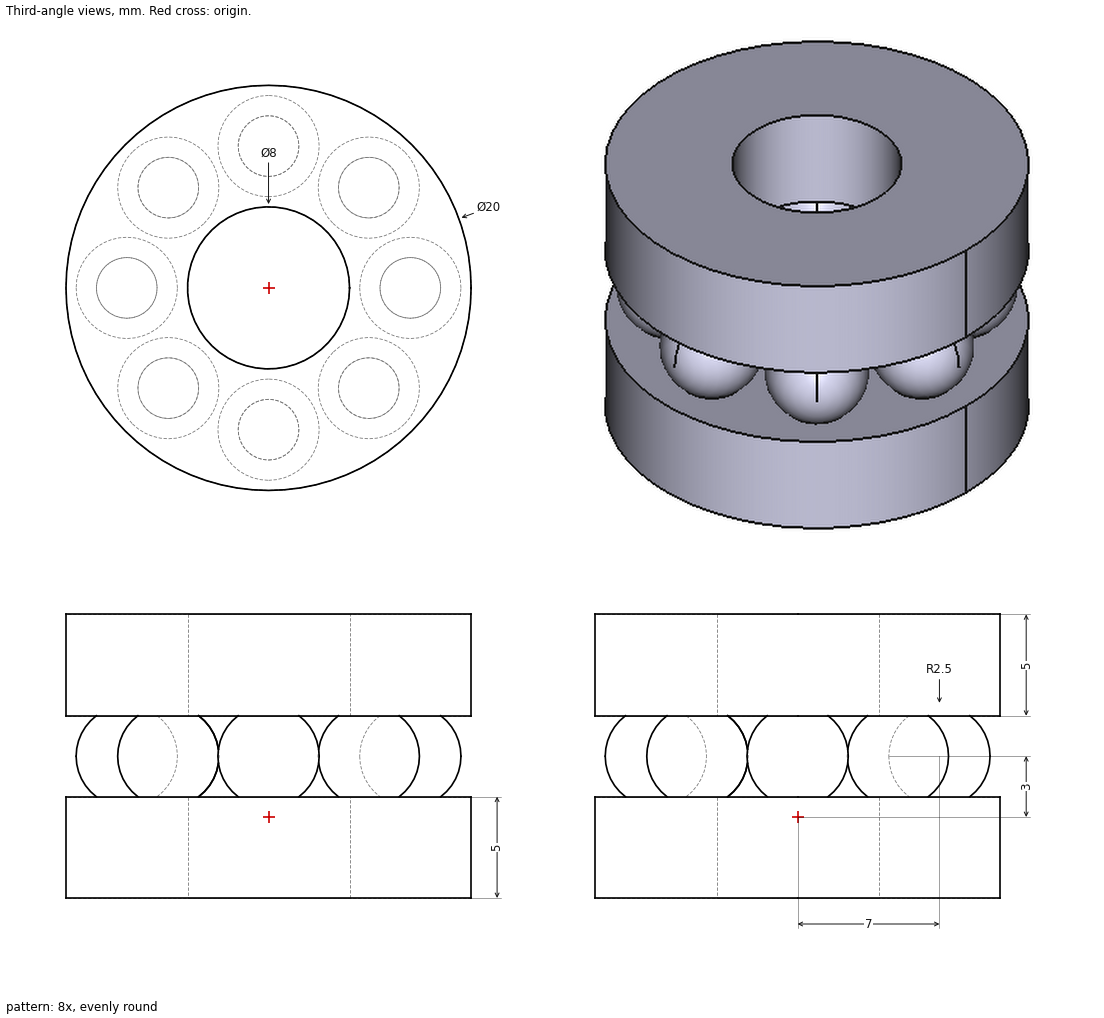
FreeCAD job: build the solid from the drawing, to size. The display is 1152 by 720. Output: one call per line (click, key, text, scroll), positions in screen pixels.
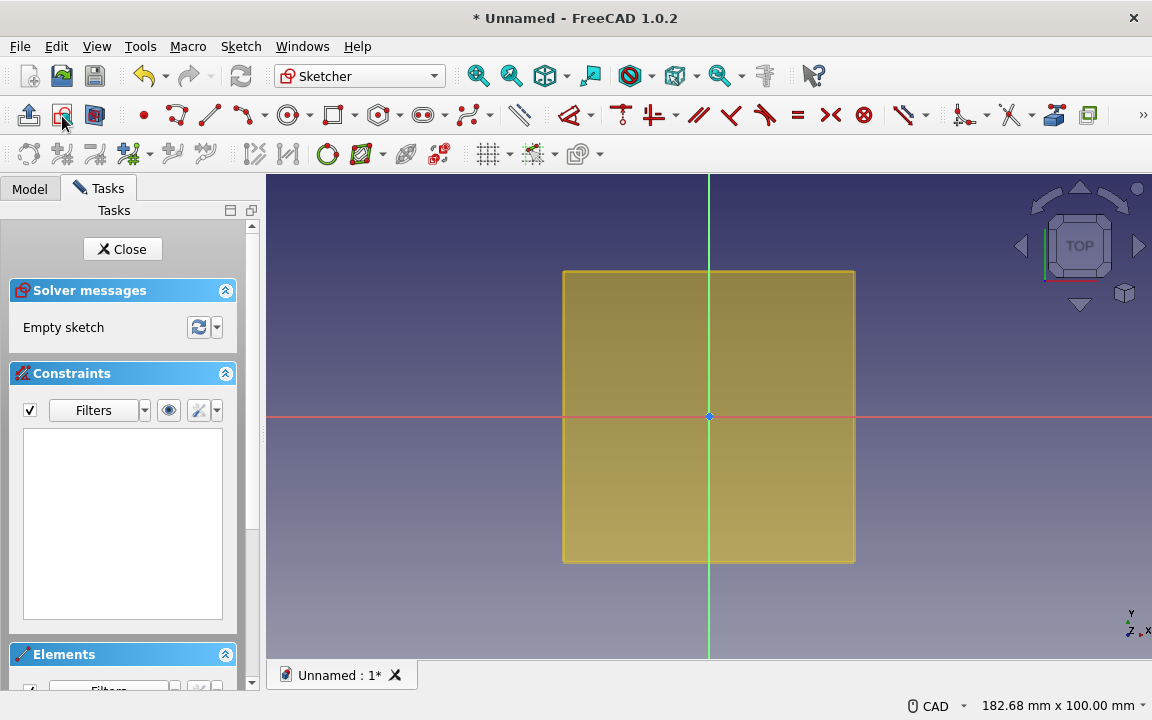
scroll(739, 416, up, 6)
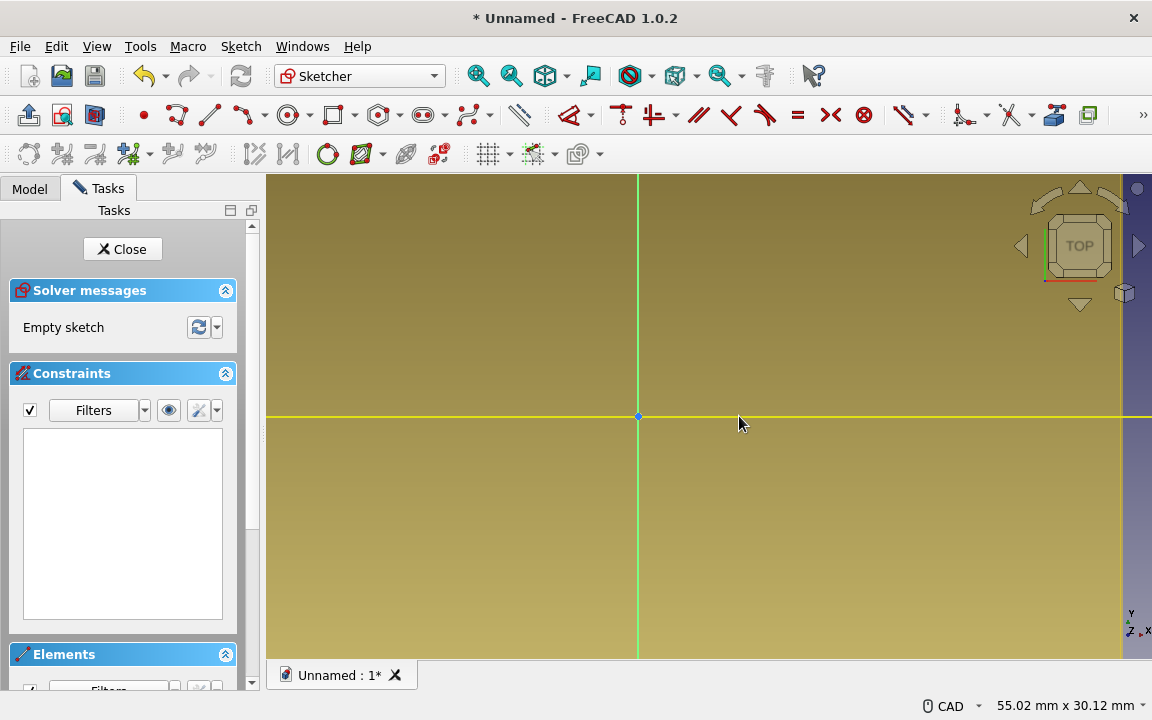
click(288, 116)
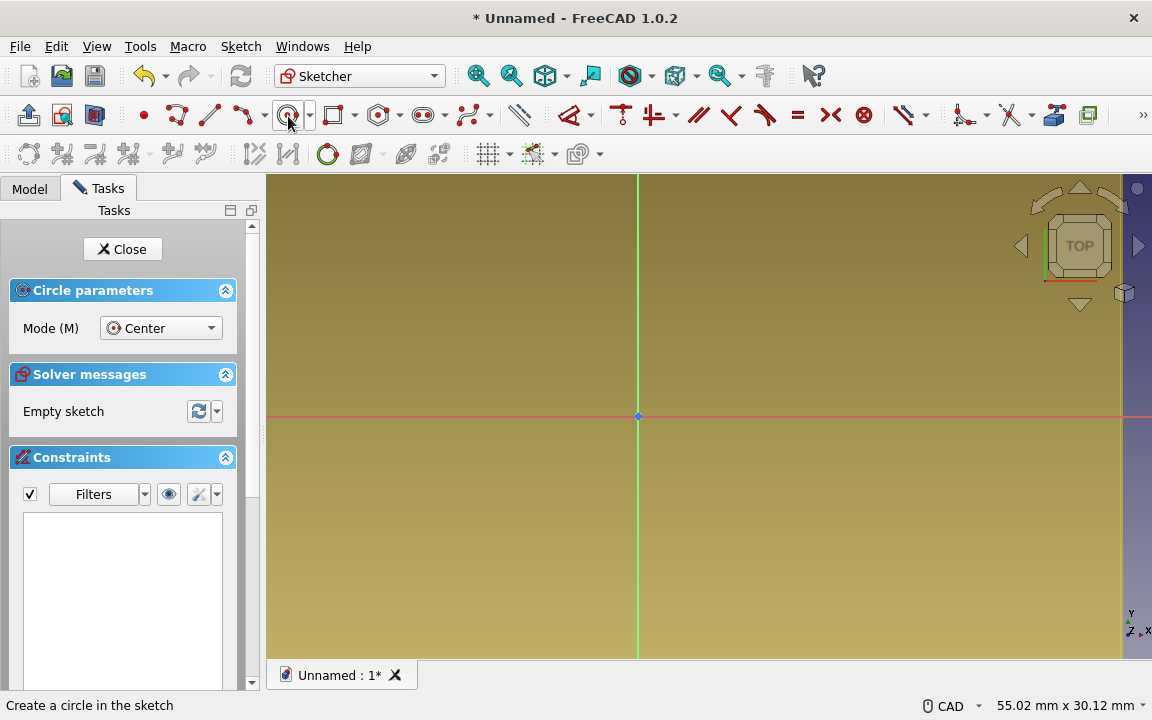
click(638, 416)
click(752, 303)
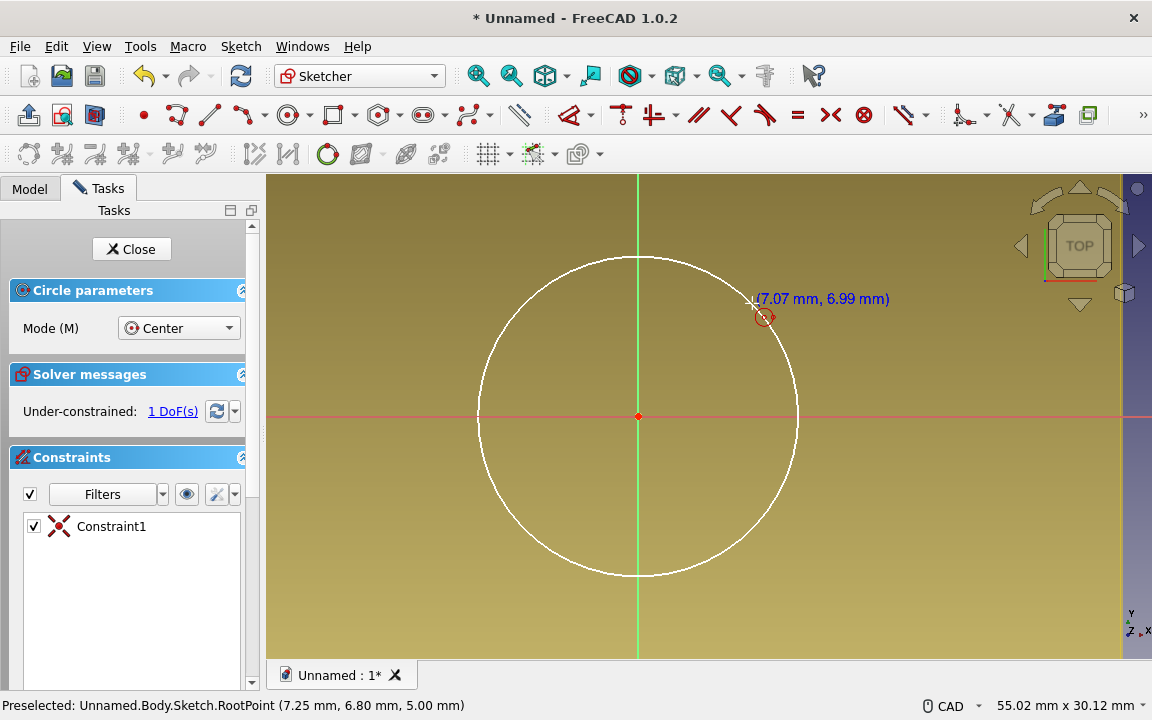
click(638, 416)
click(684, 371)
key(Escape)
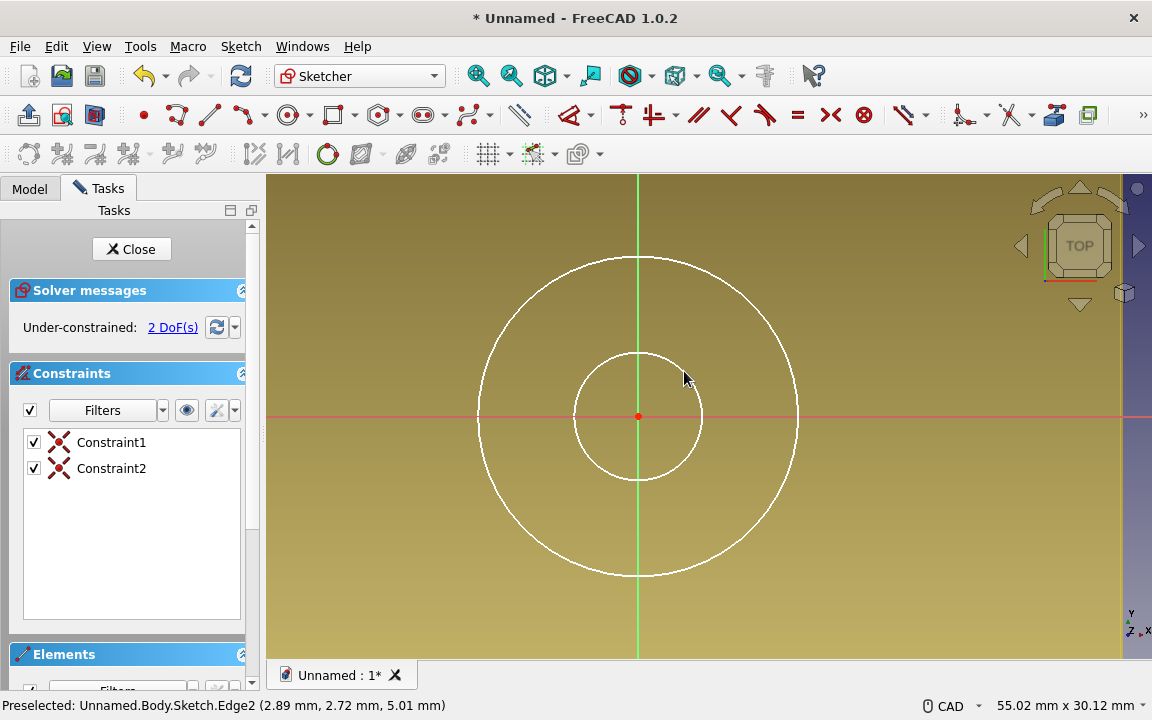
click(568, 116)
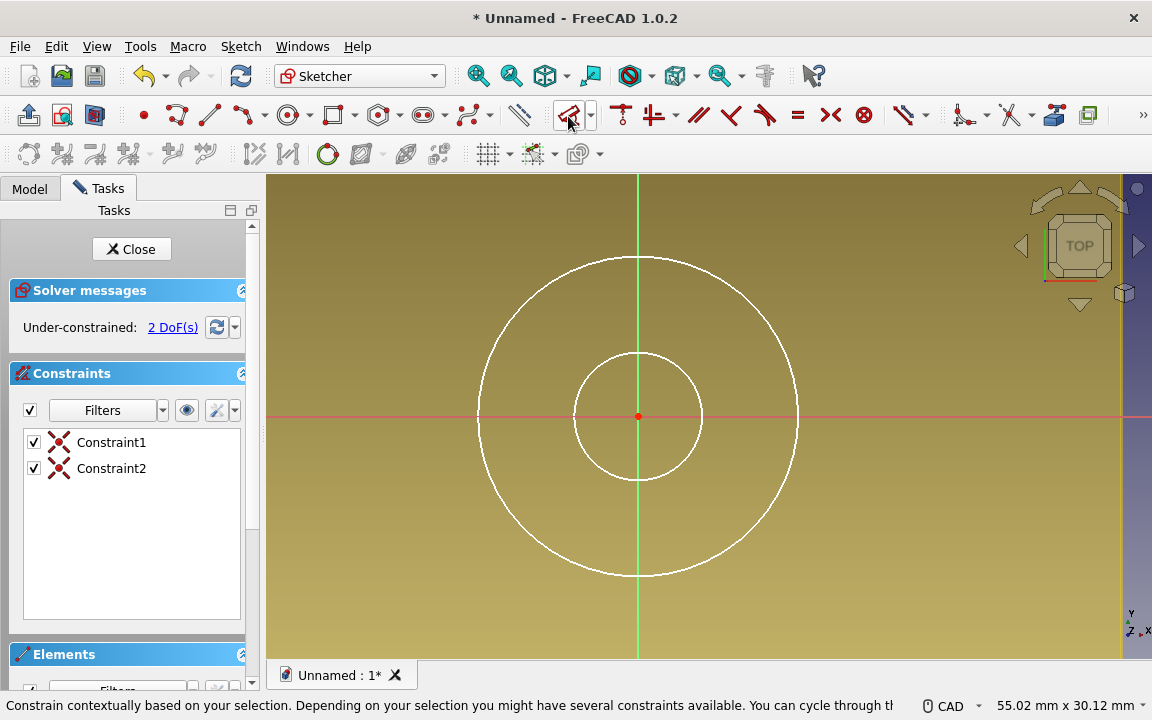
click(751, 303)
click(774, 280)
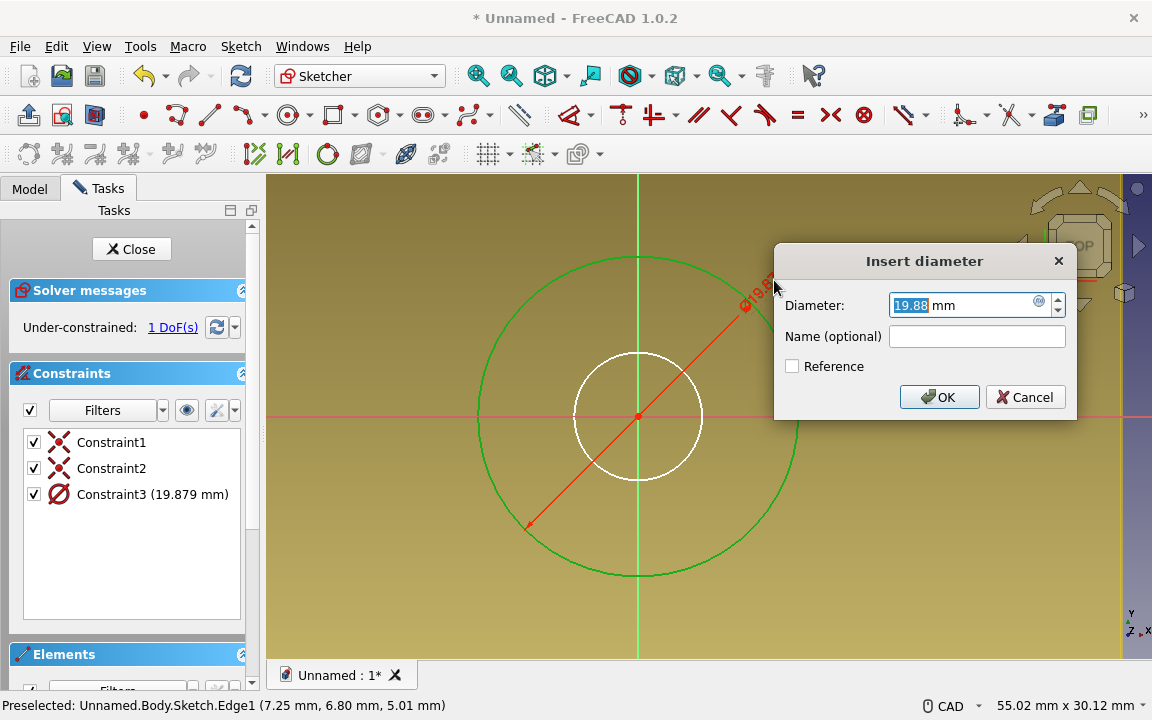
text(20)
key(Return)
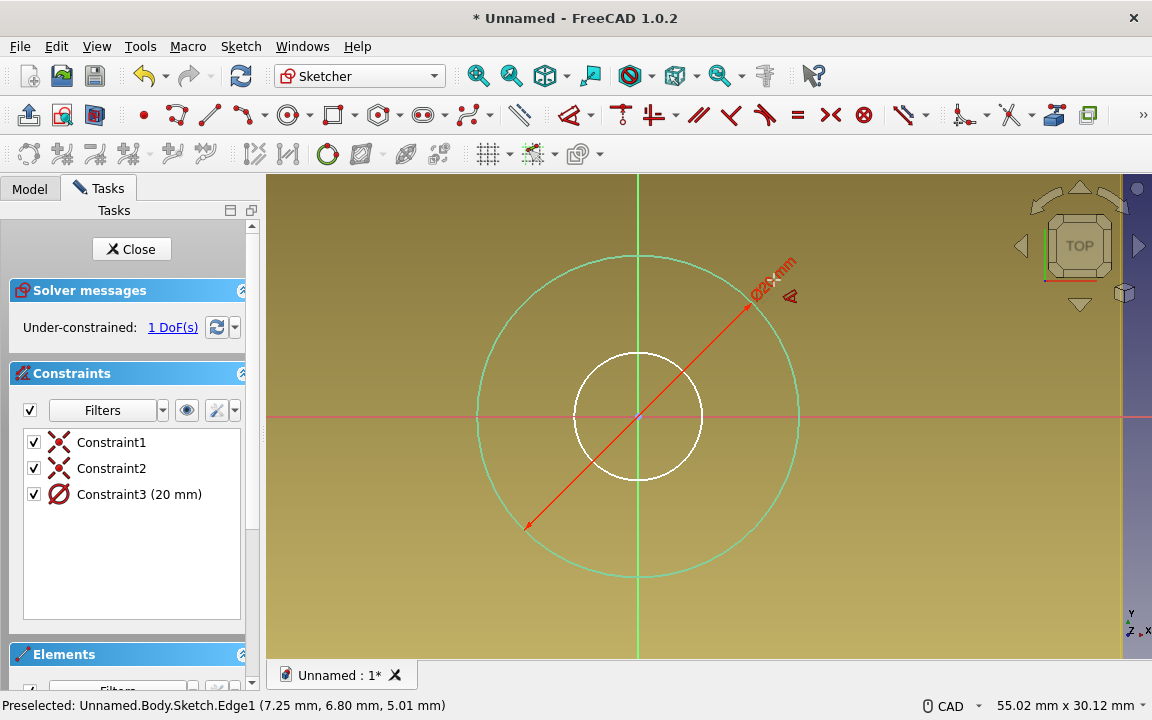
click(683, 371)
click(705, 348)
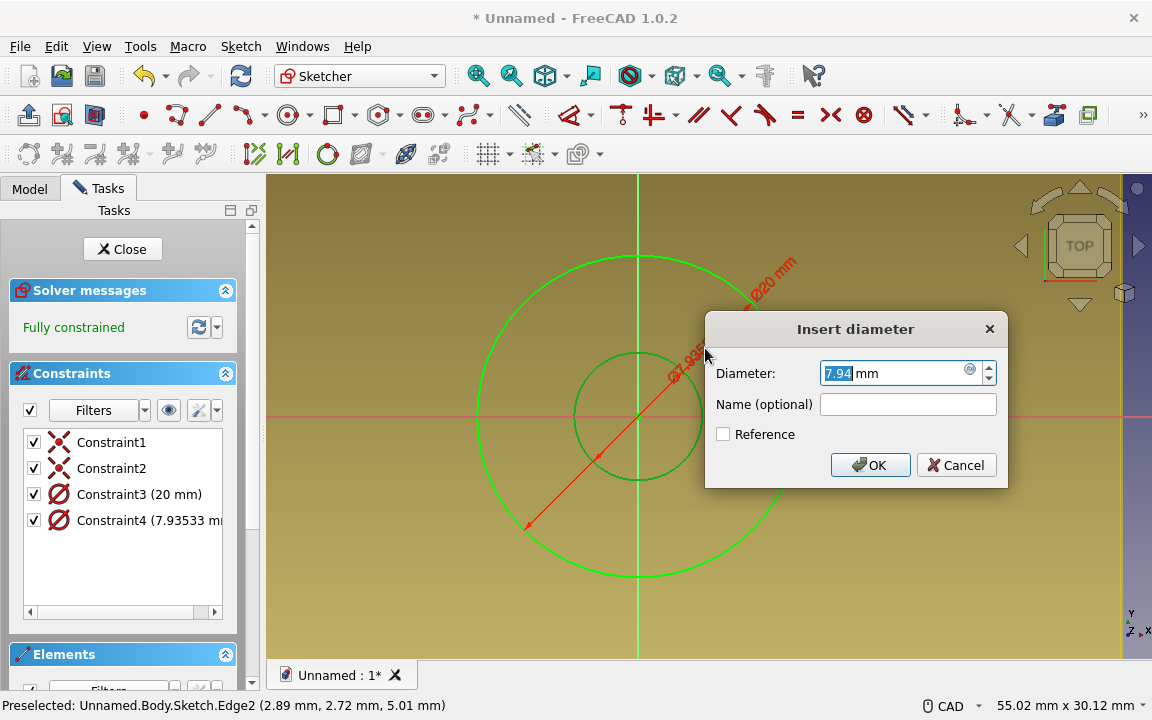
text(8)
key(Return)
key(Escape)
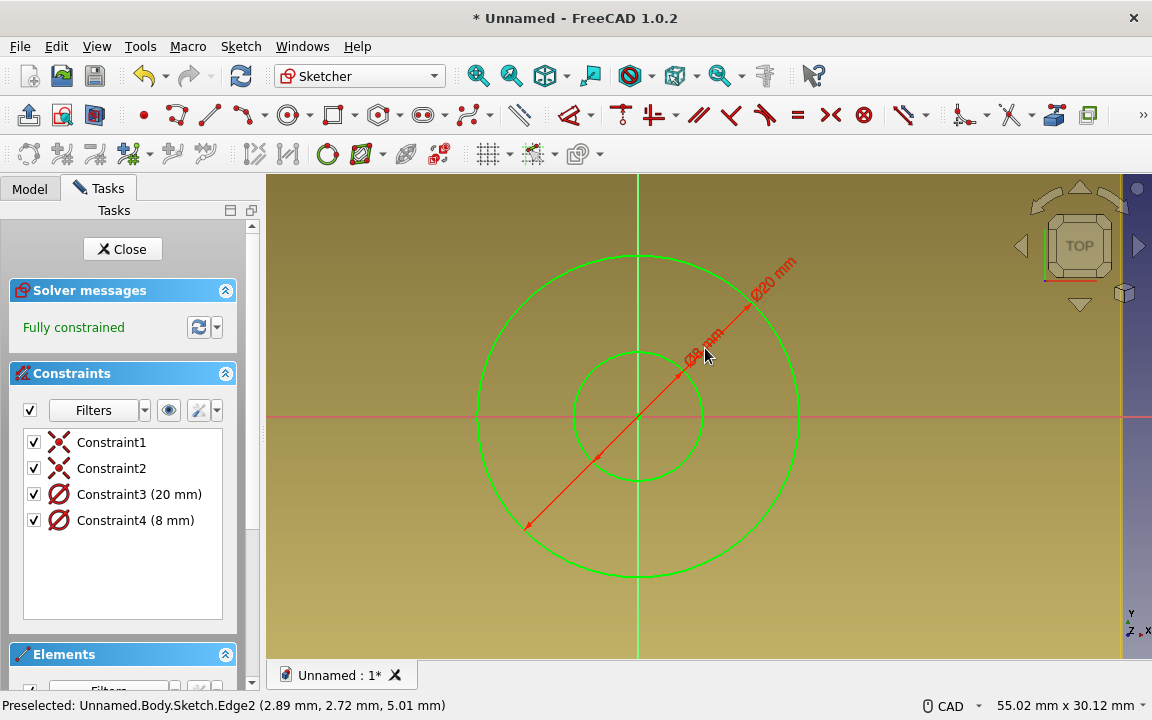
click(123, 249)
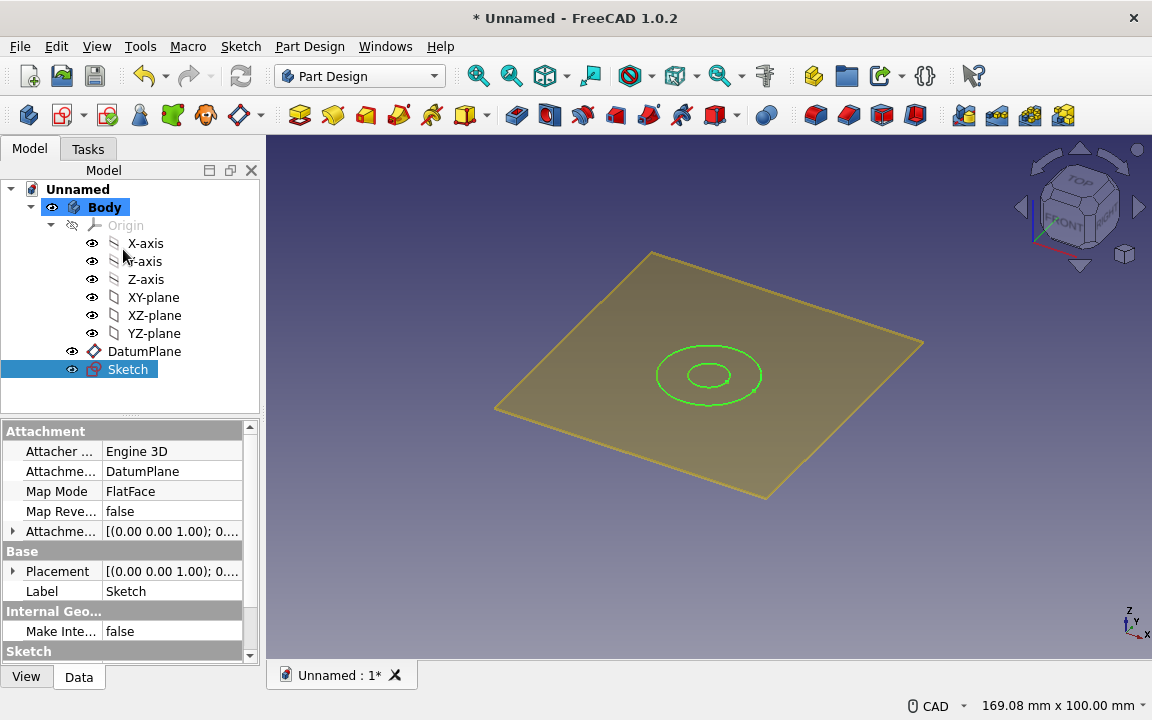
click(300, 116)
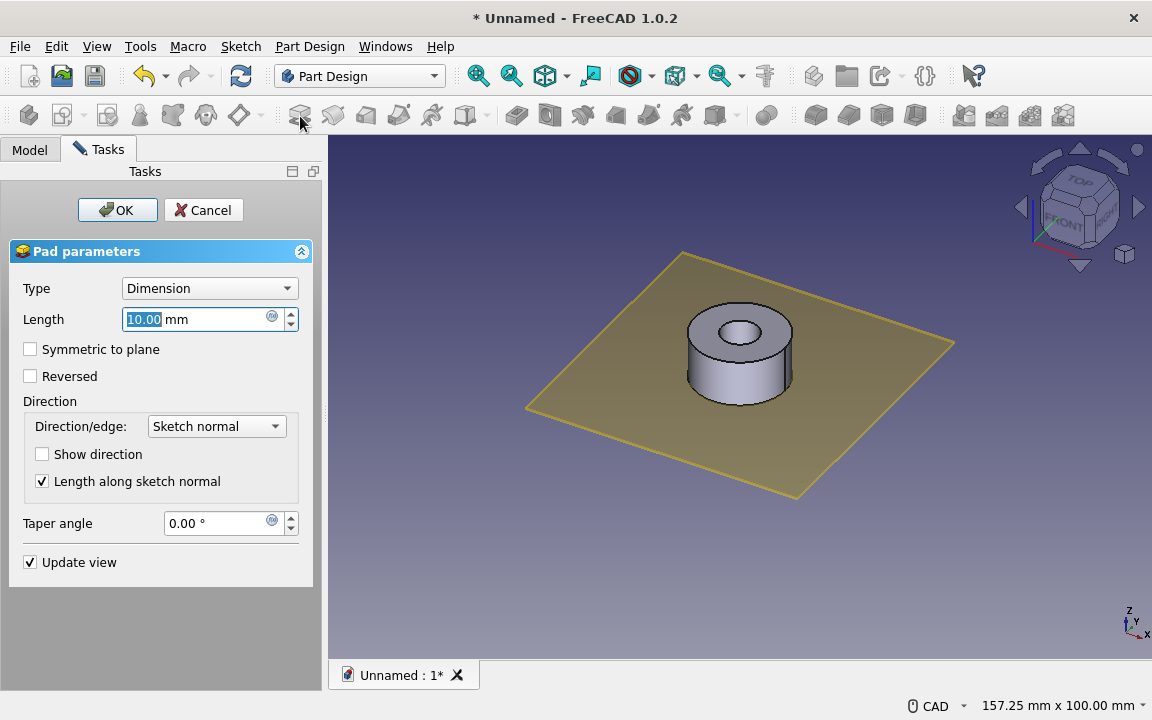
text(5)
key(Tab)